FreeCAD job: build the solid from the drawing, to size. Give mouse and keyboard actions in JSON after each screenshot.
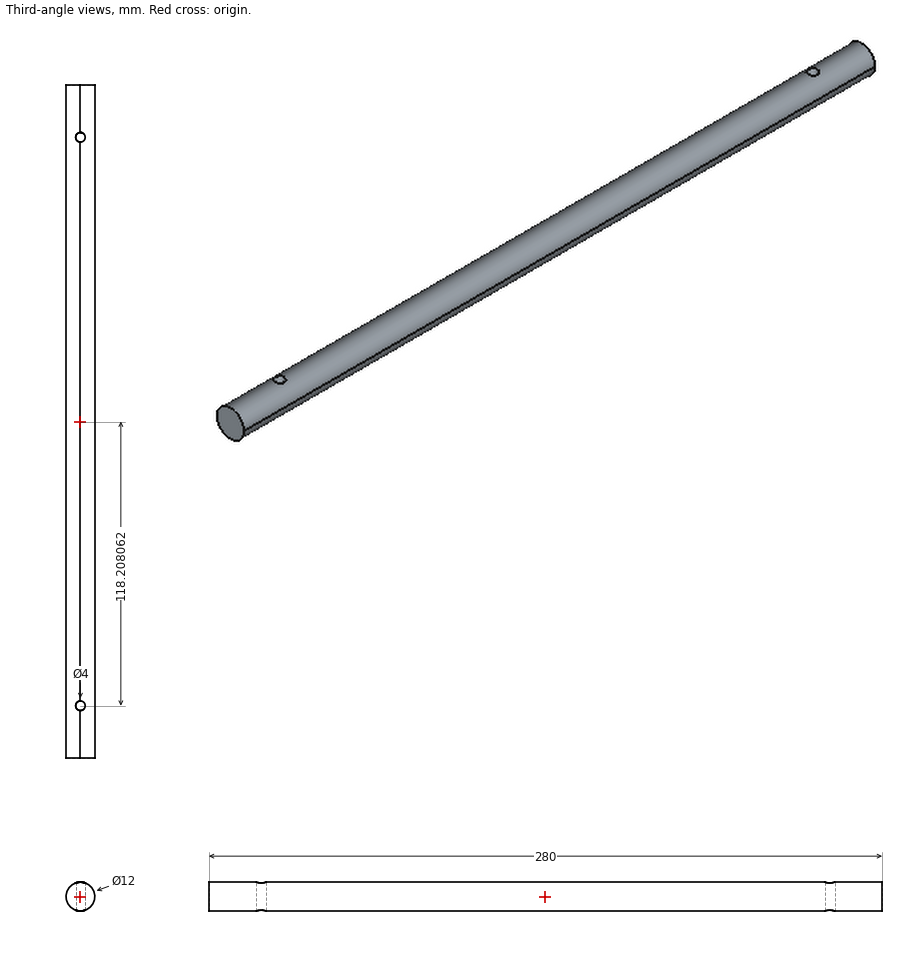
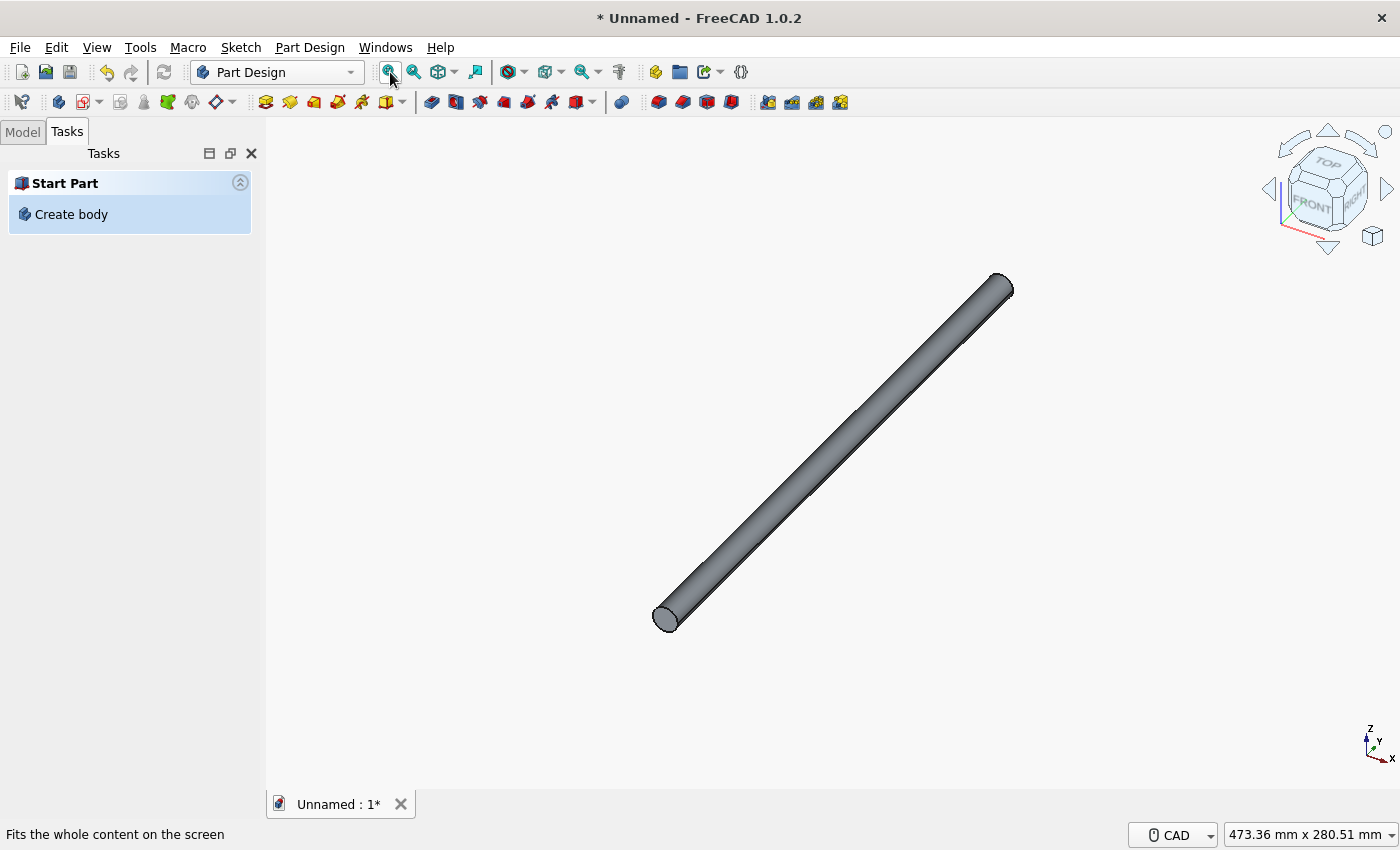
{"action": "left_click", "coordinate": [23, 131]}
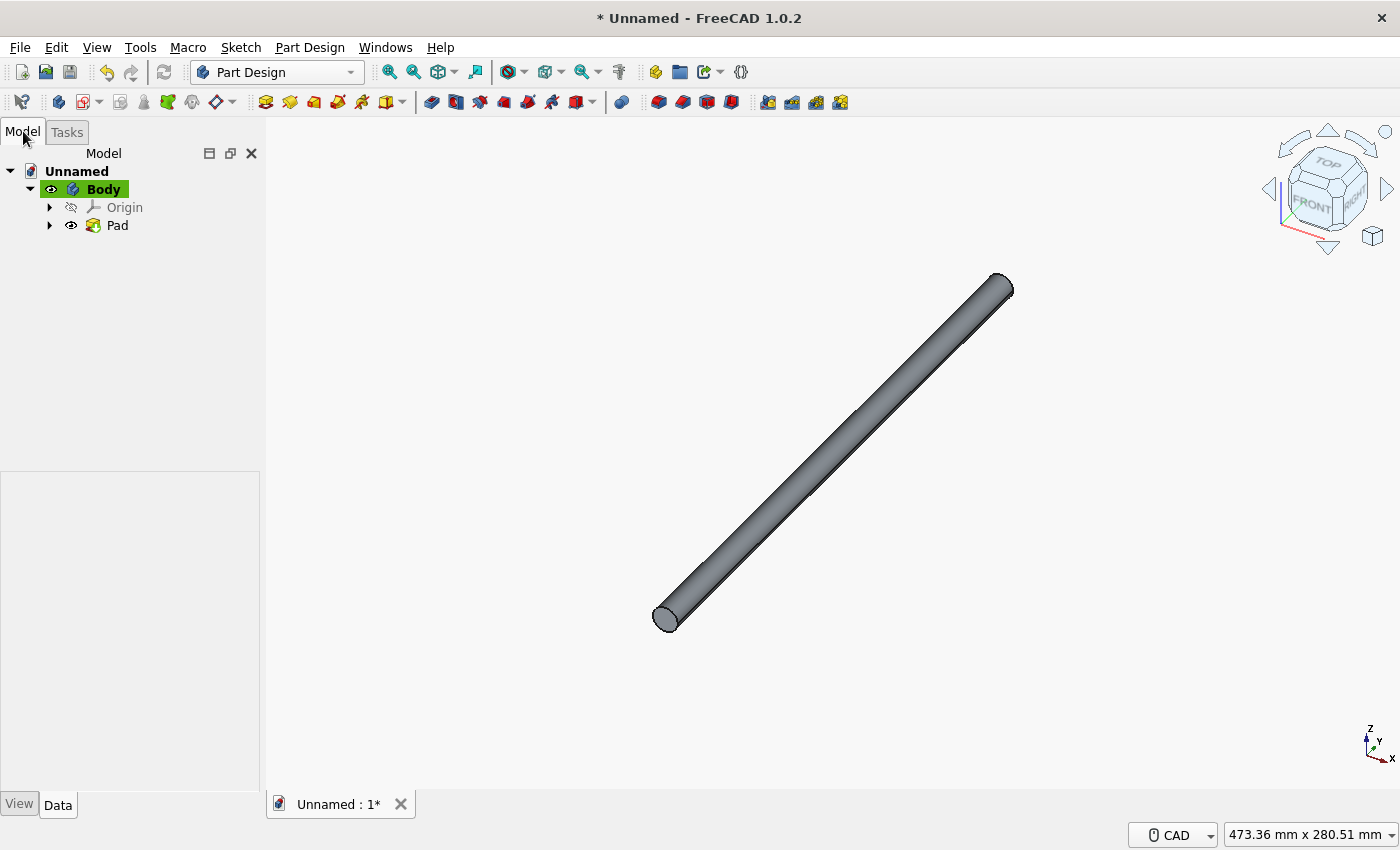
{"action": "left_click", "coordinate": [50, 207]}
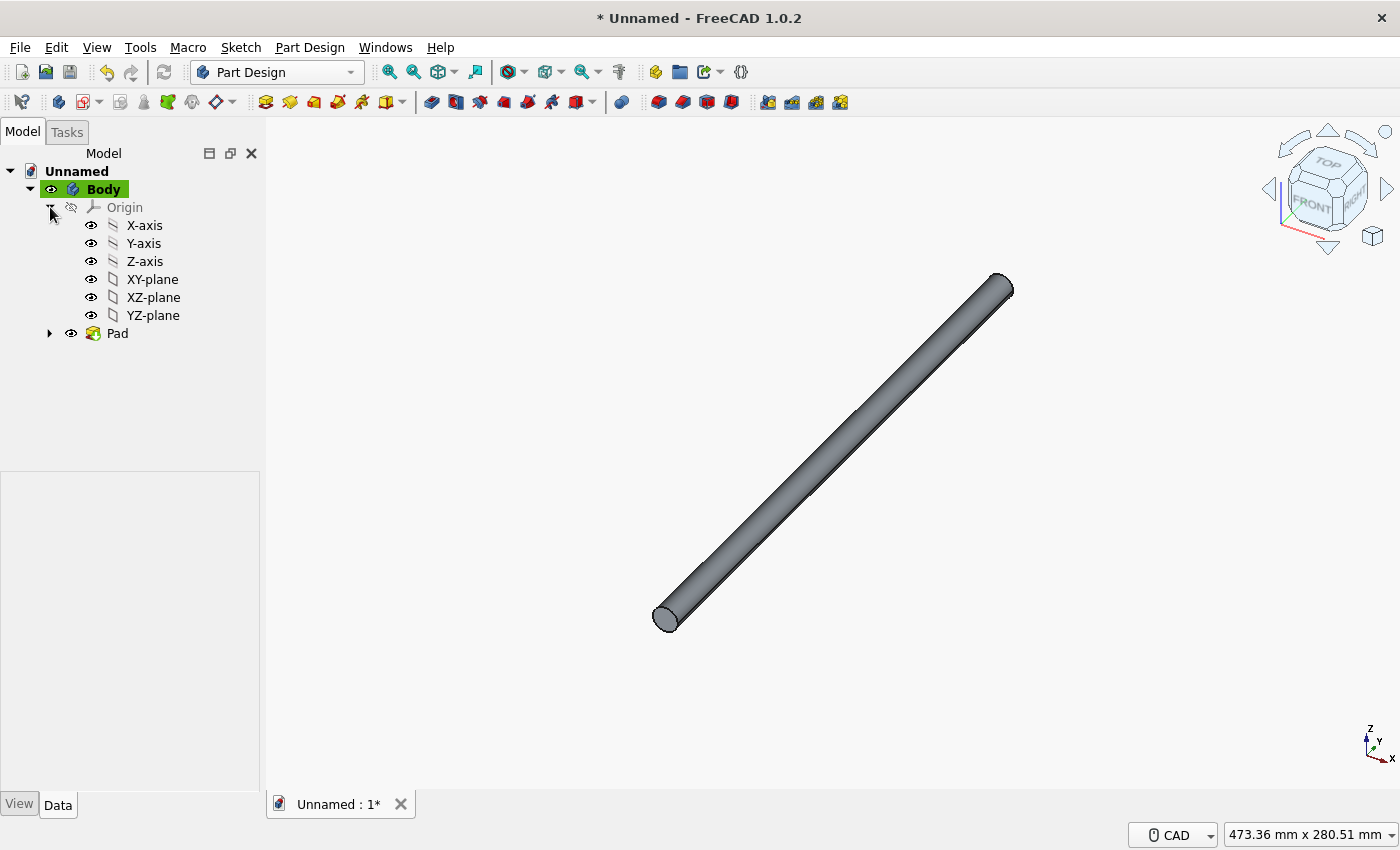
{"action": "left_click", "coordinate": [136, 279]}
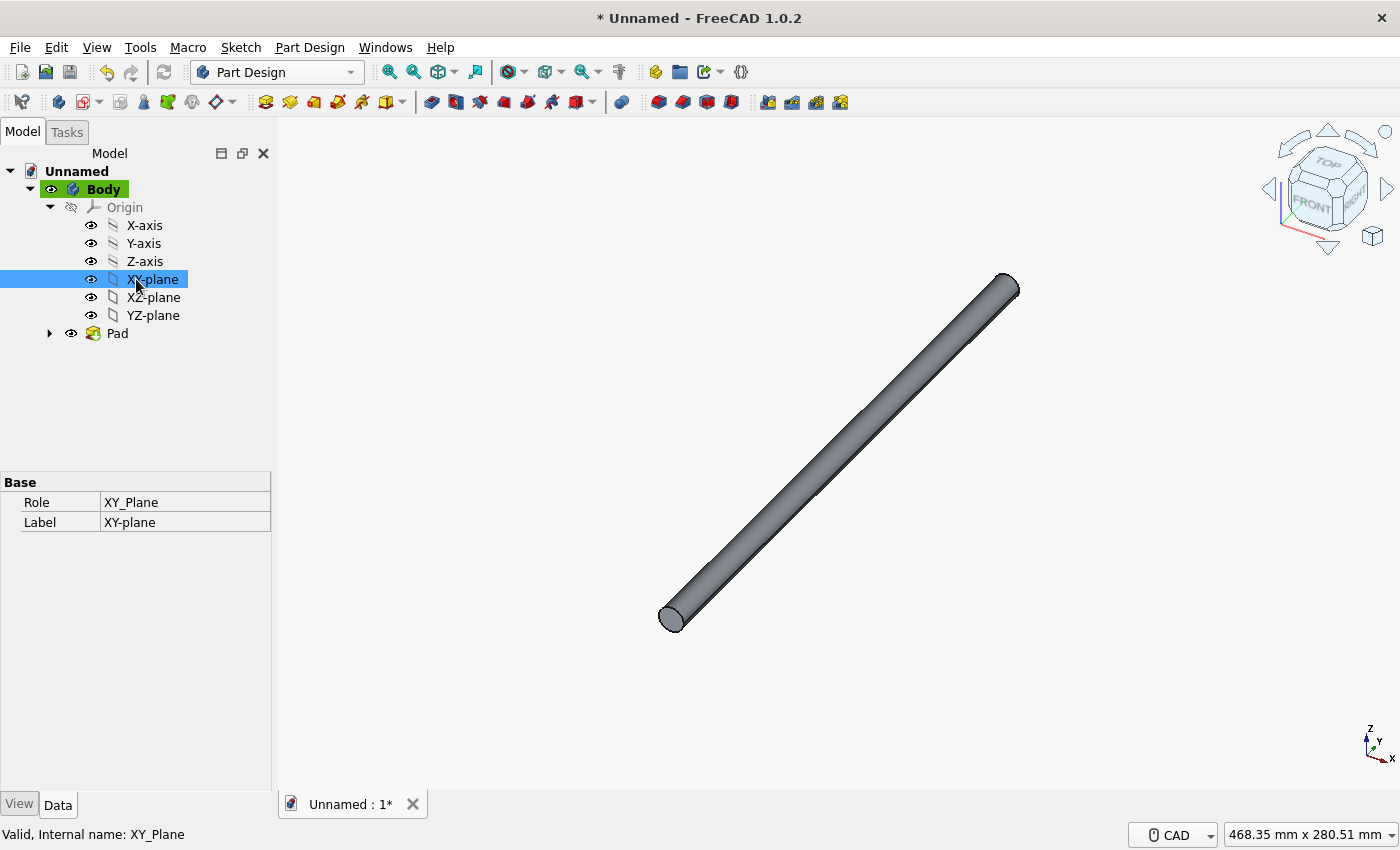
{"action": "left_click", "coordinate": [216, 102]}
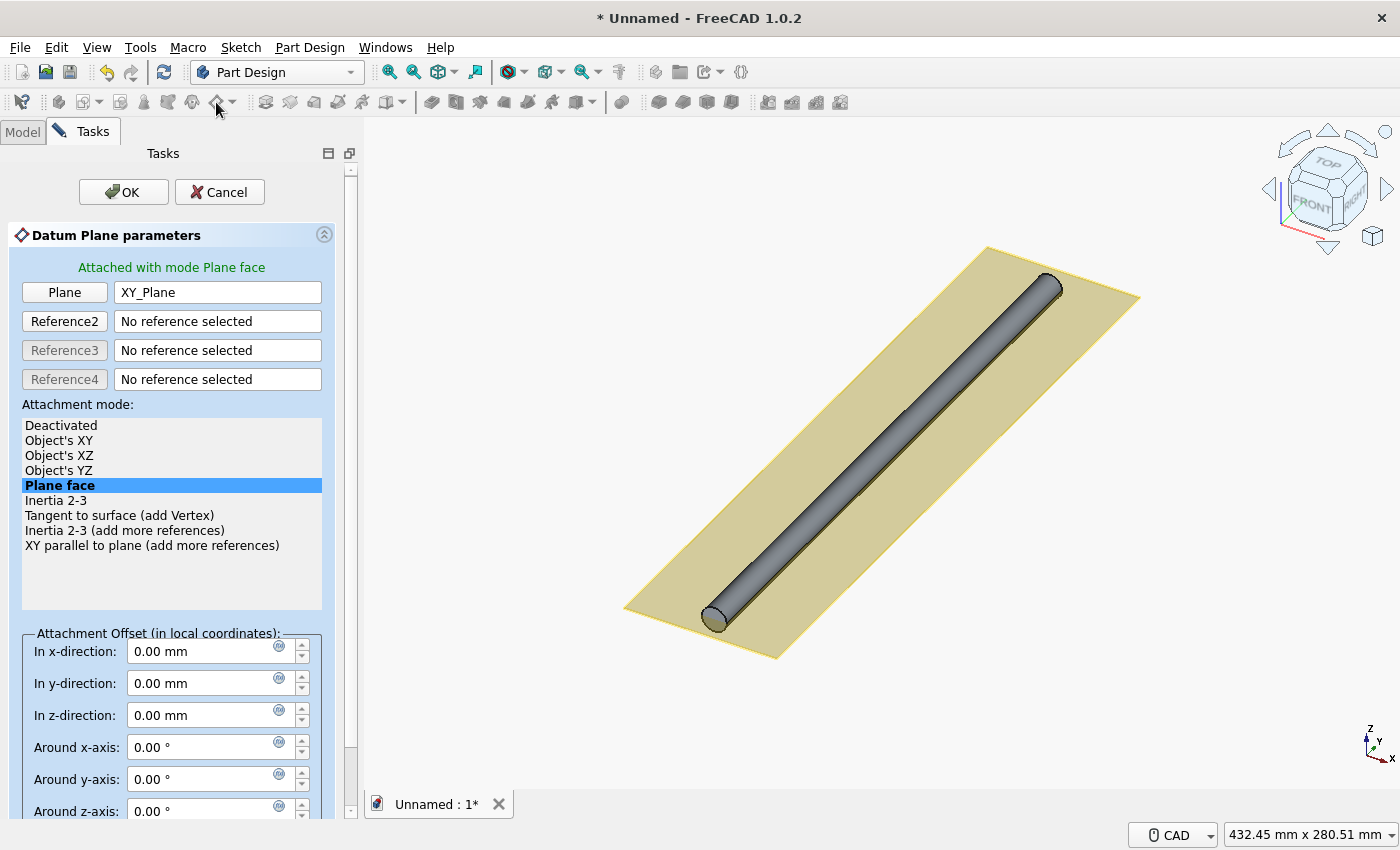
{"action": "triple_click", "coordinate": [210, 715]}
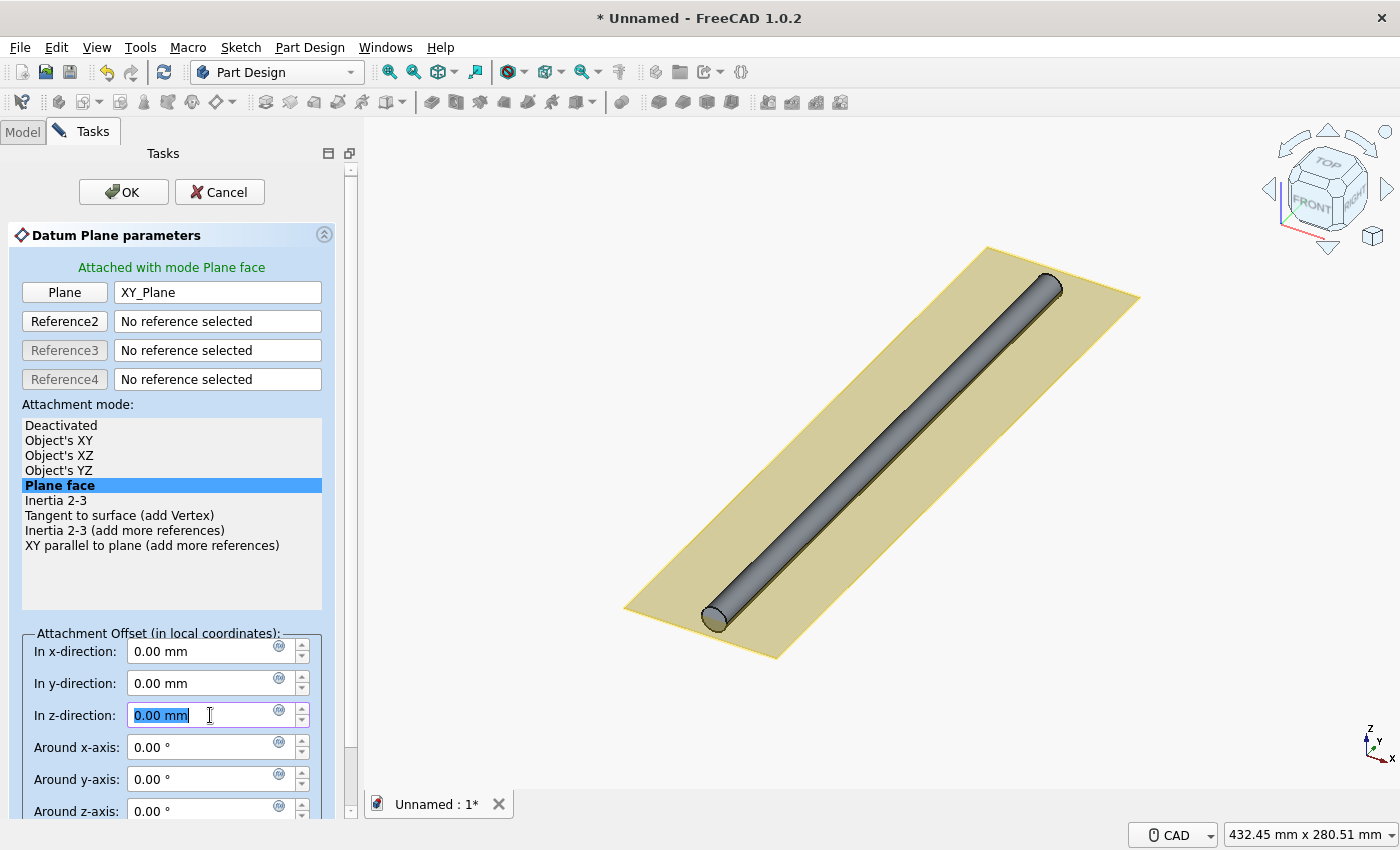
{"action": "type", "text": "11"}
{"action": "key", "text": "Tab"}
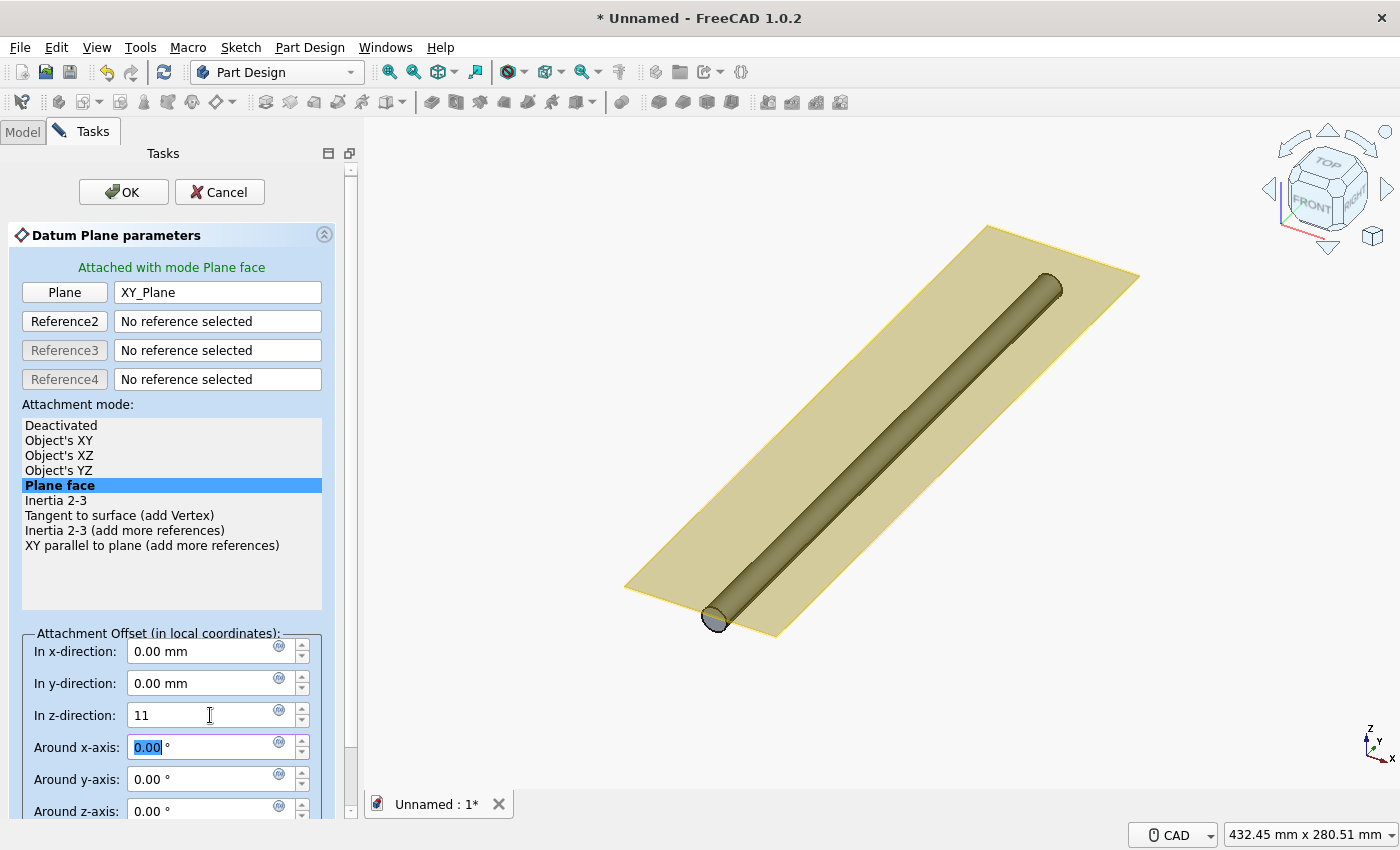
{"action": "left_click", "coordinate": [124, 192]}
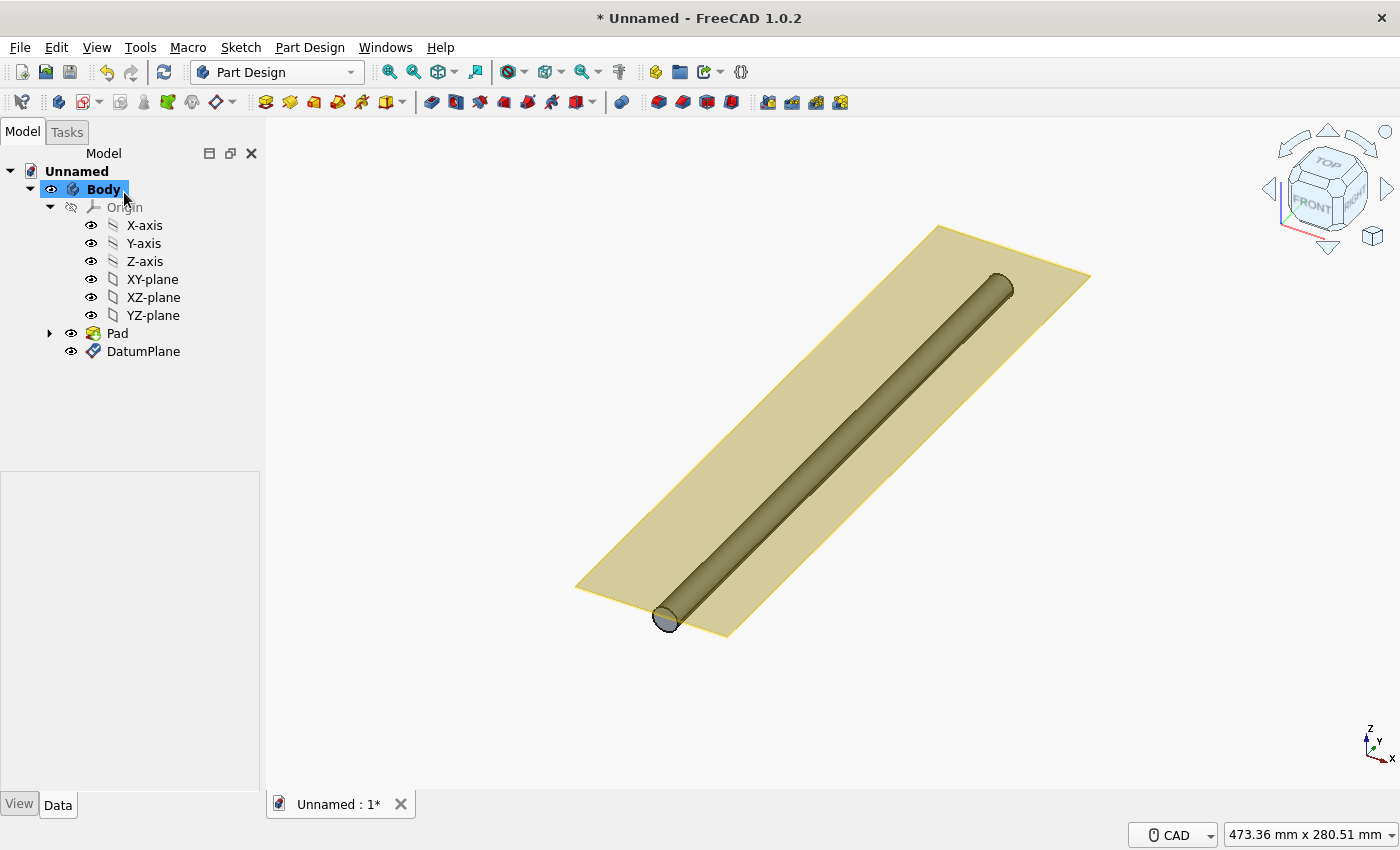
{"action": "left_click", "coordinate": [116, 351]}